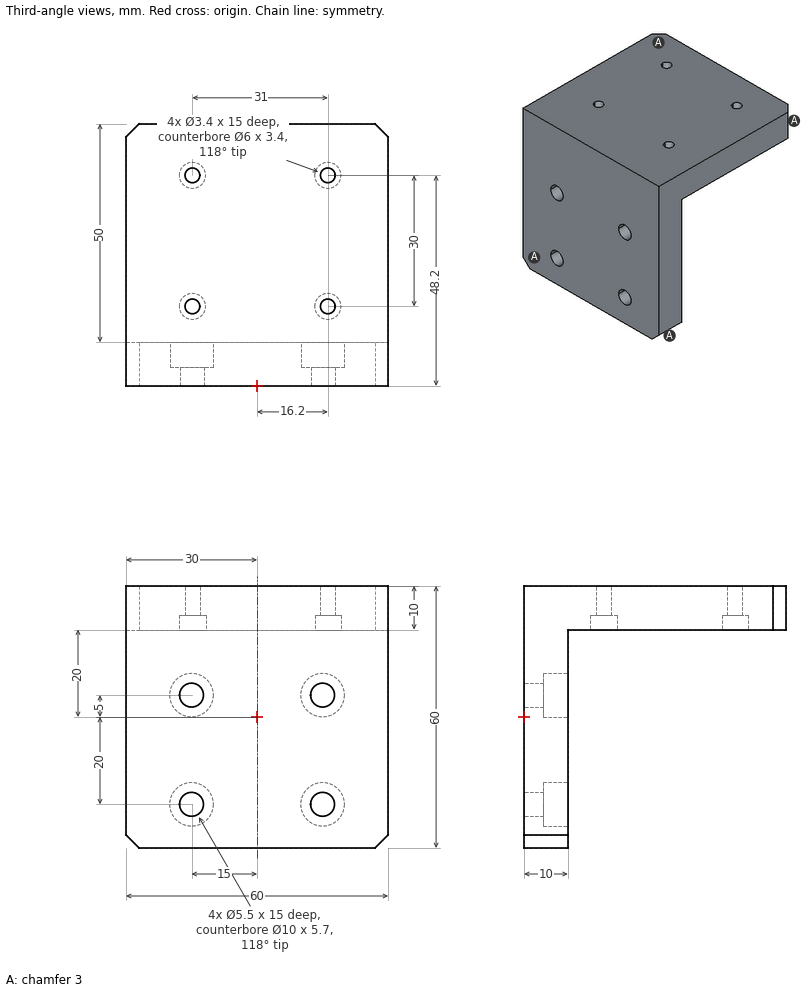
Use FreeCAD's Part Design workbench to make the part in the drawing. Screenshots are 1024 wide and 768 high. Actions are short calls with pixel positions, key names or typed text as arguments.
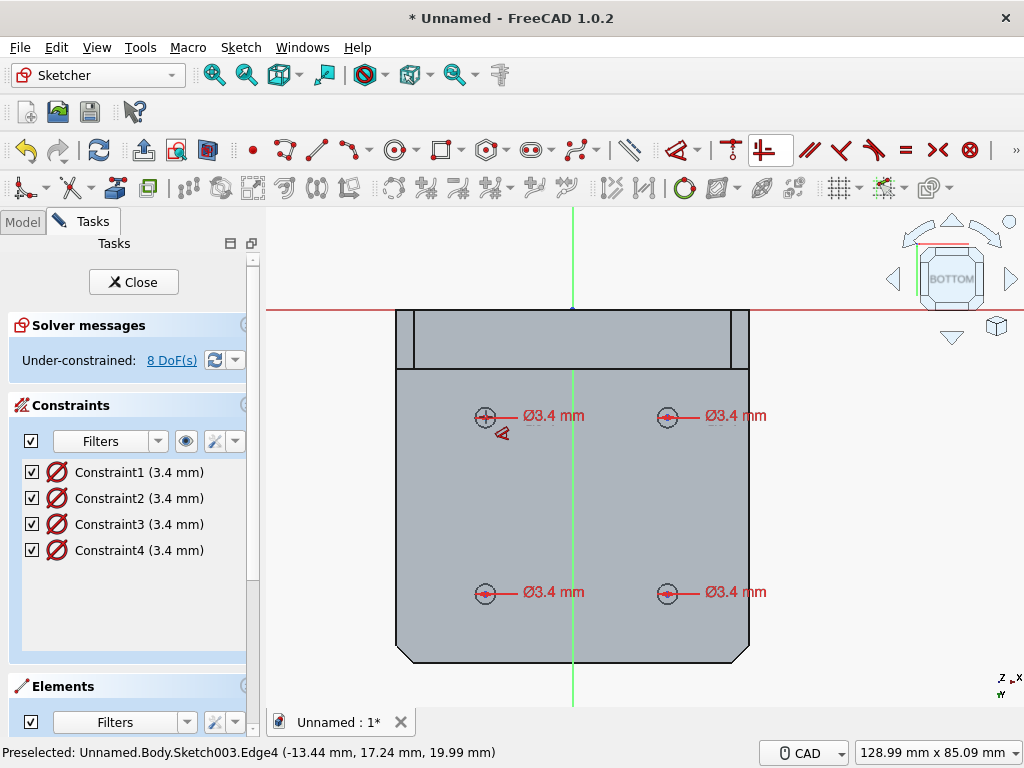
click(668, 594)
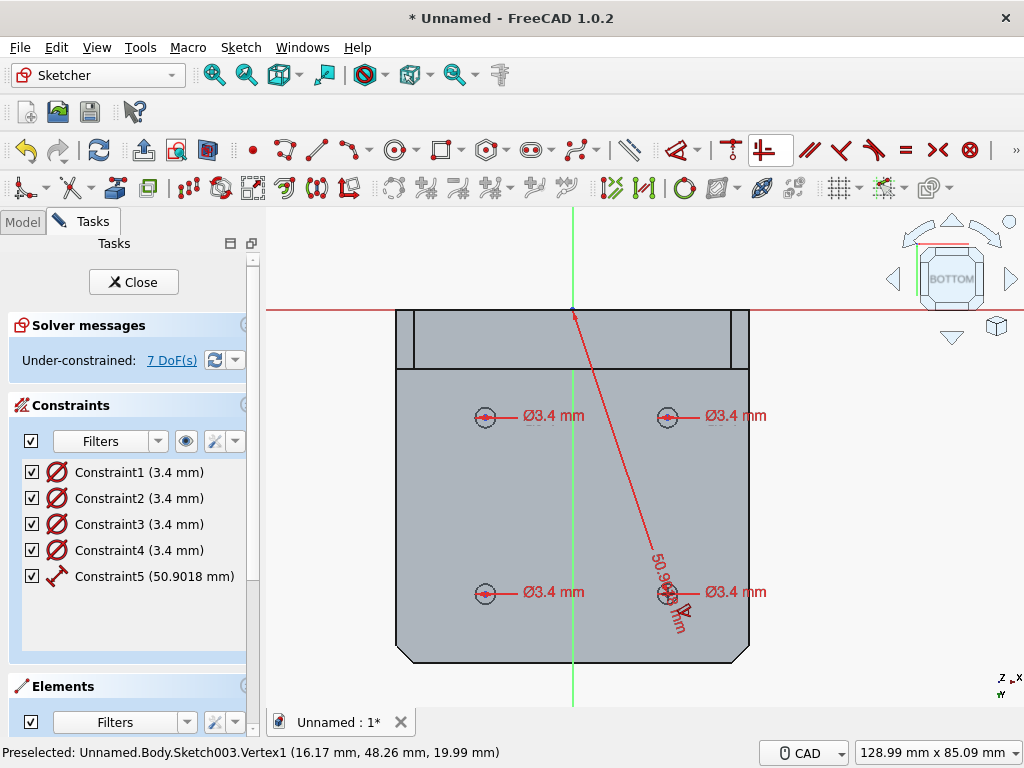
click(485, 594)
click(535, 628)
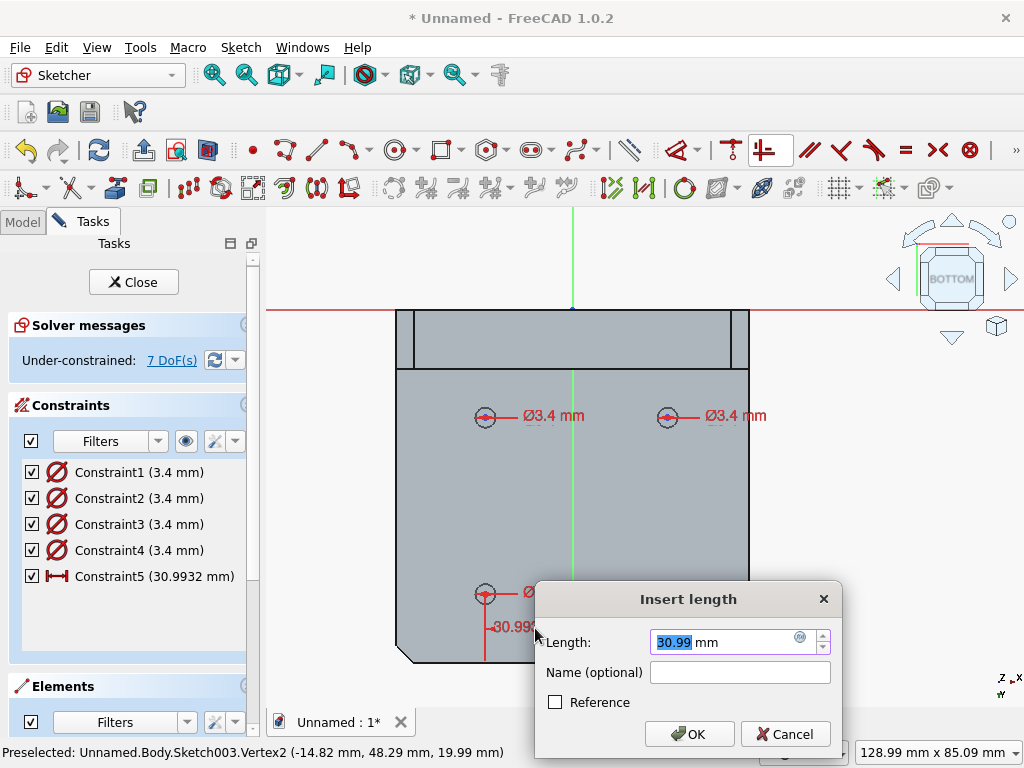
text(31)
key(Return)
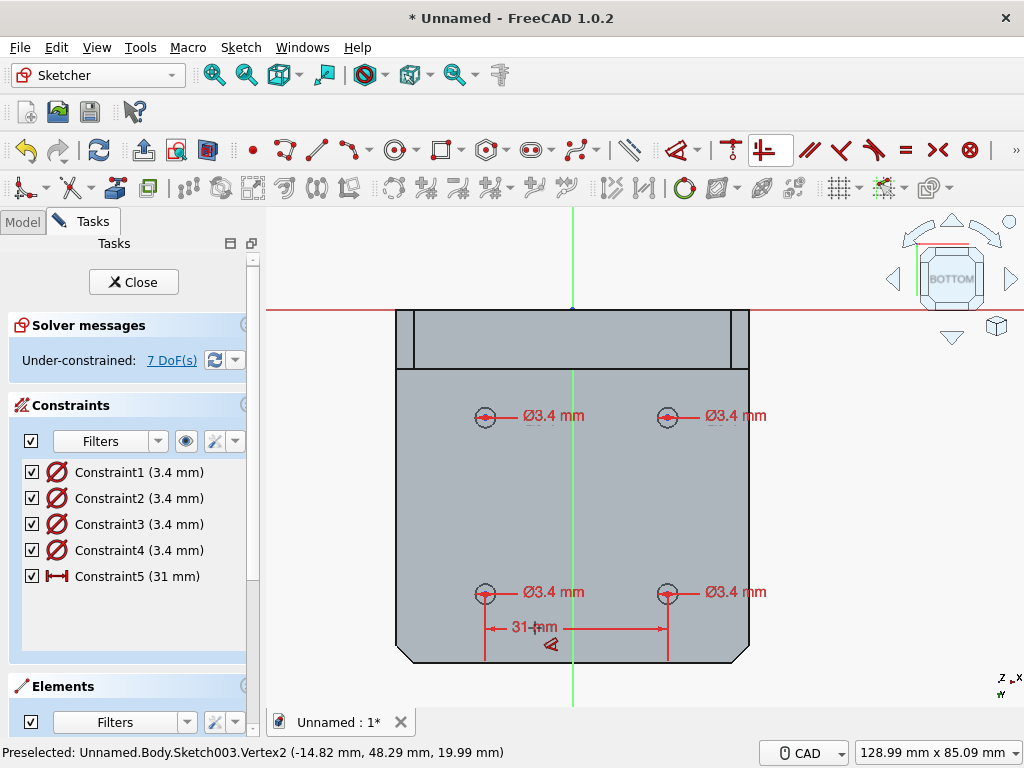
click(485, 594)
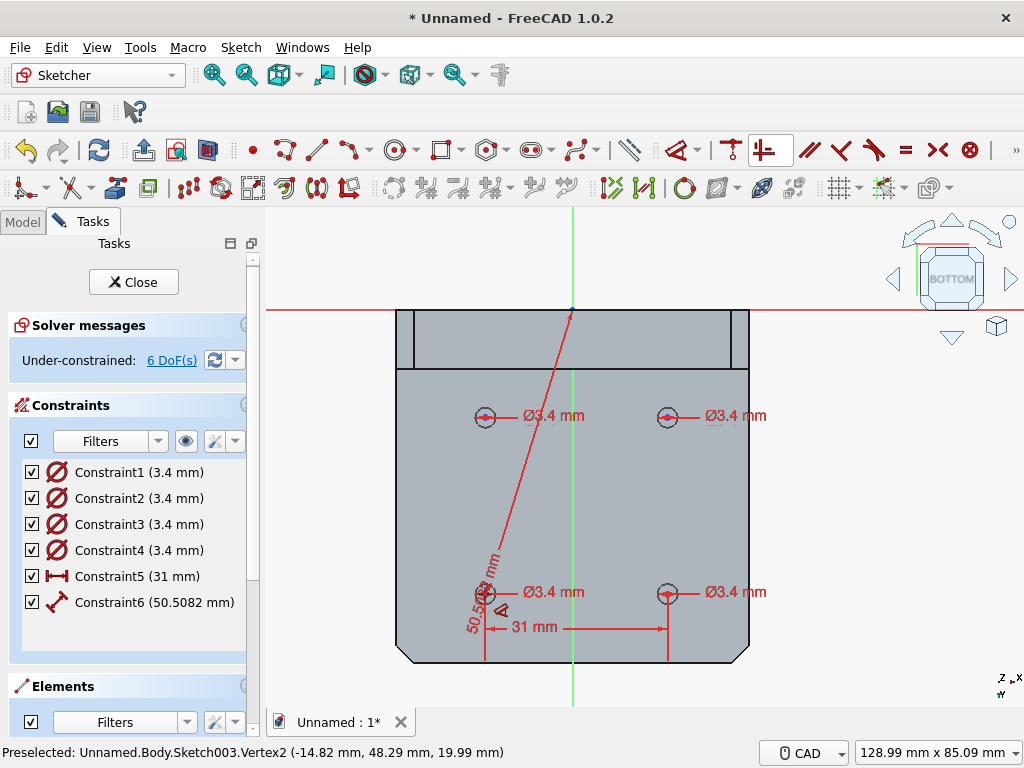
click(668, 418)
click(618, 628)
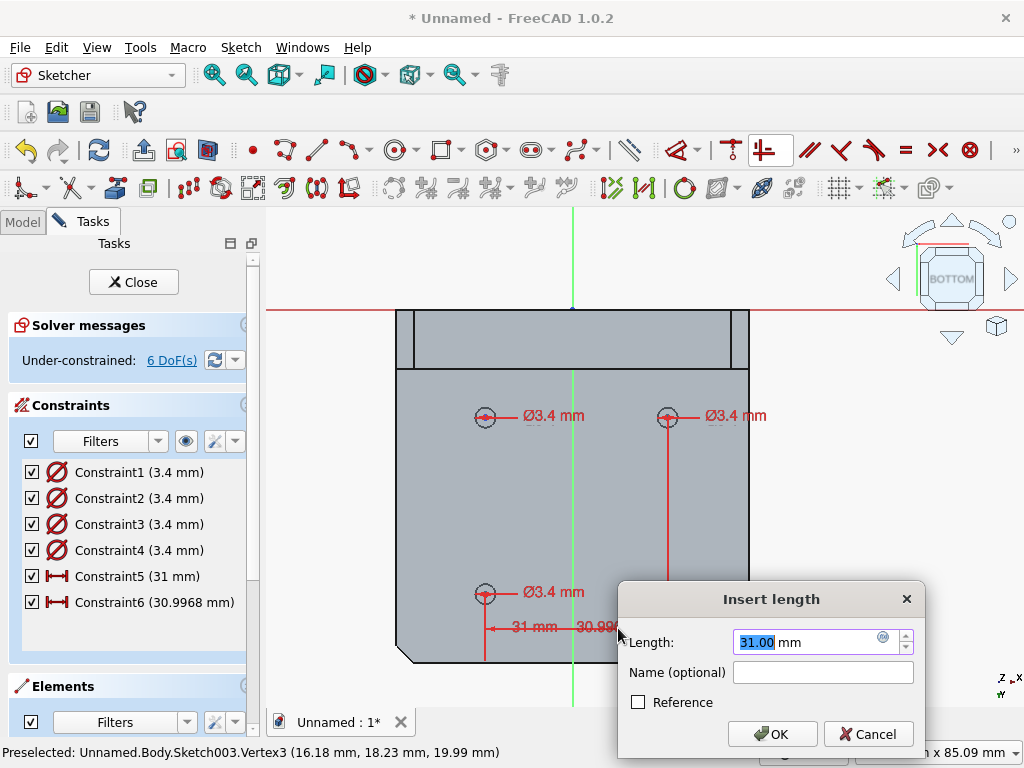
text(31)
key(Return)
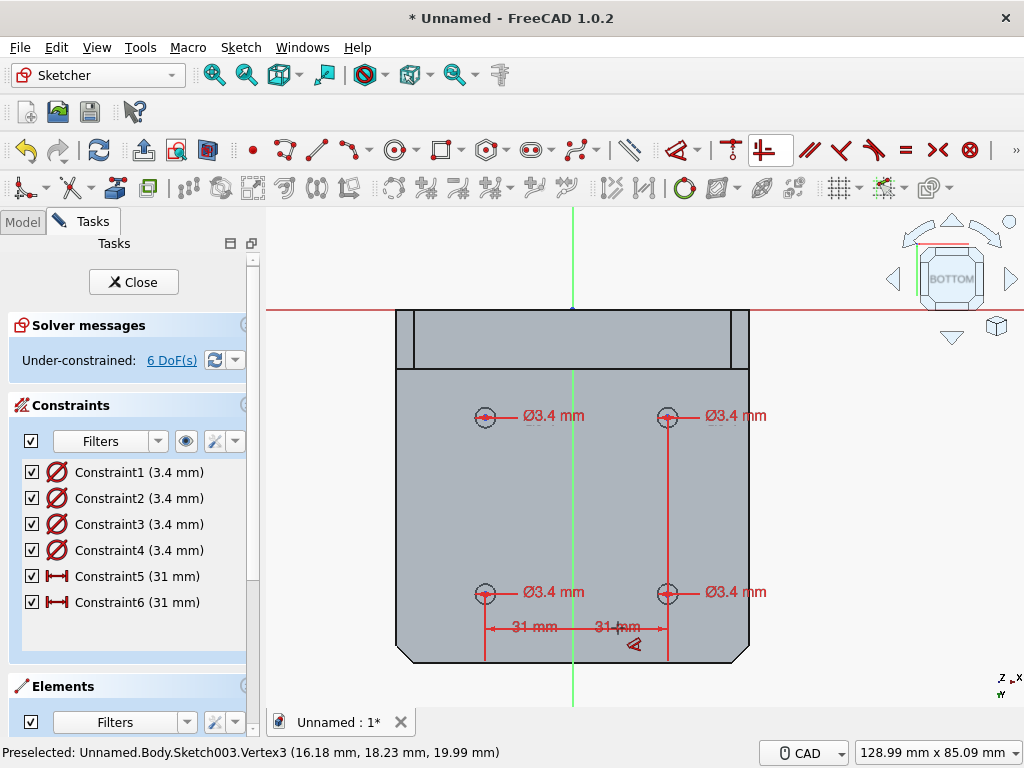
click(668, 594)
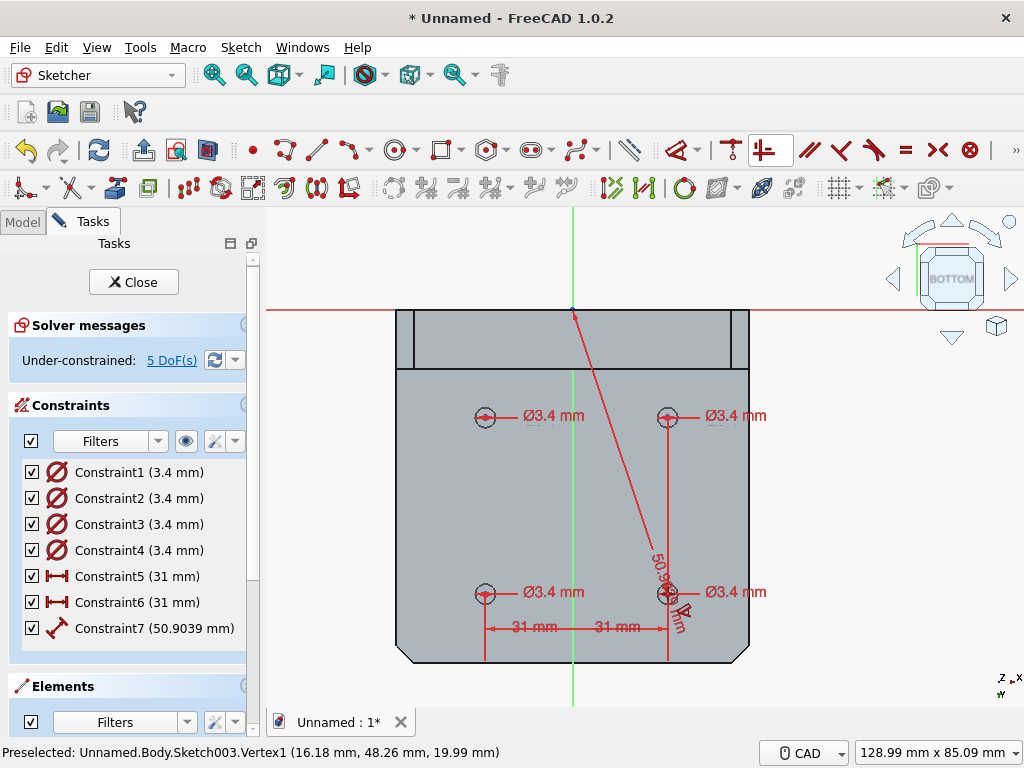
click(668, 418)
click(702, 506)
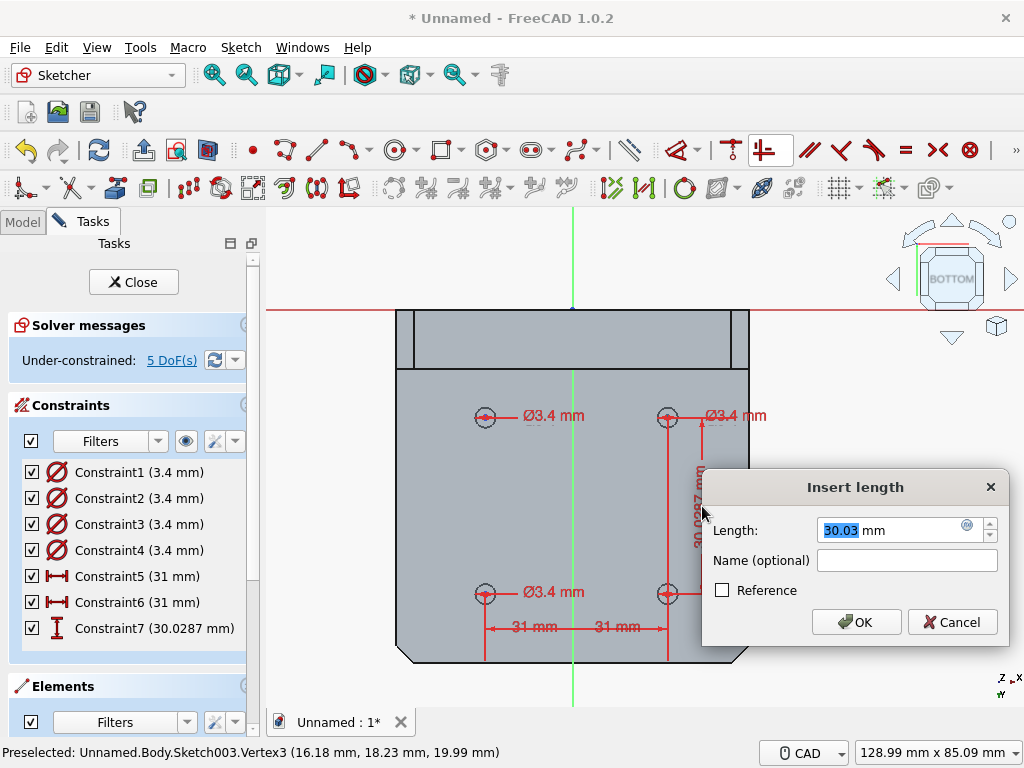
text(30)
key(Return)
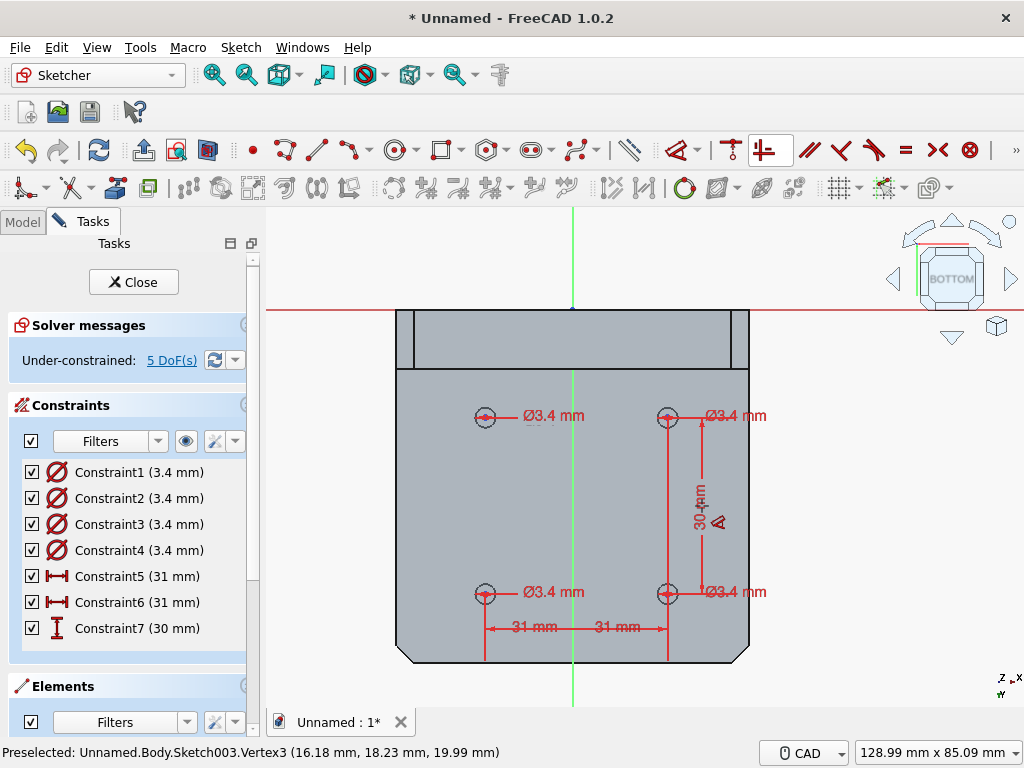
click(485, 594)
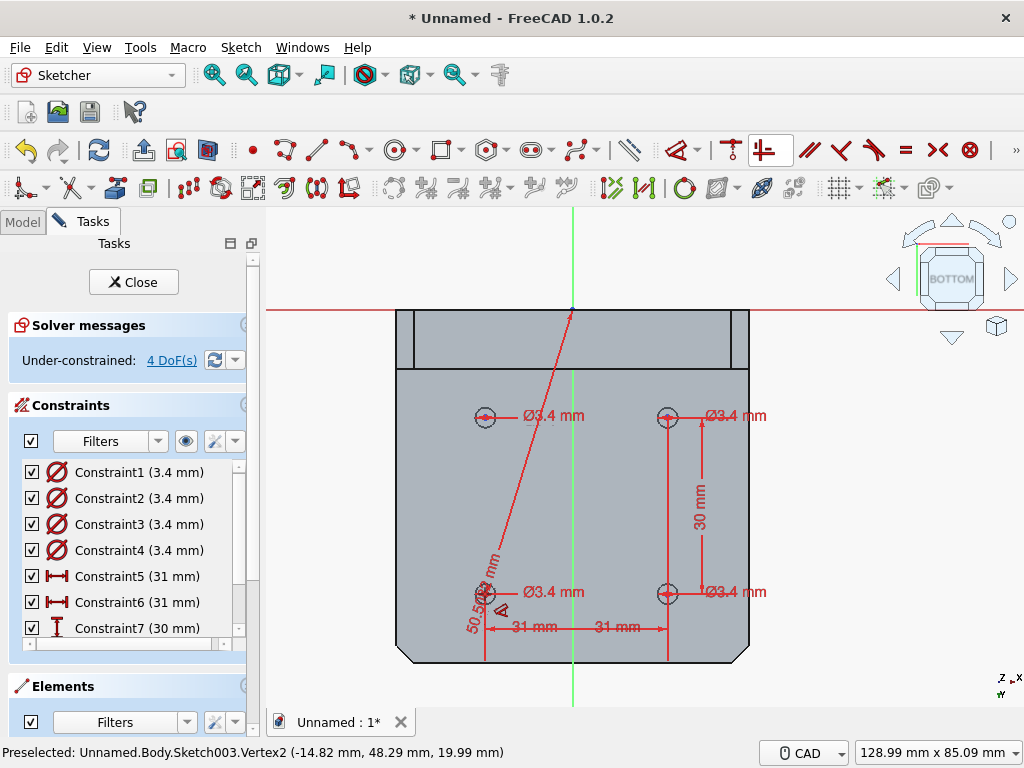
click(668, 418)
click(451, 506)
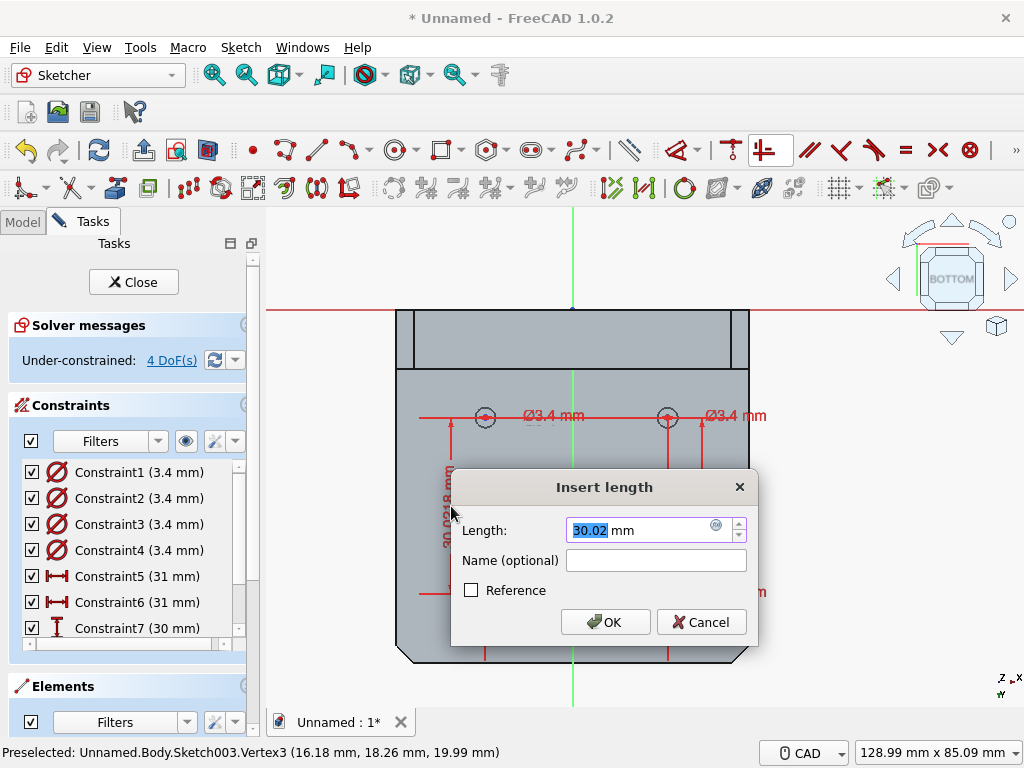
text(30)
key(Return)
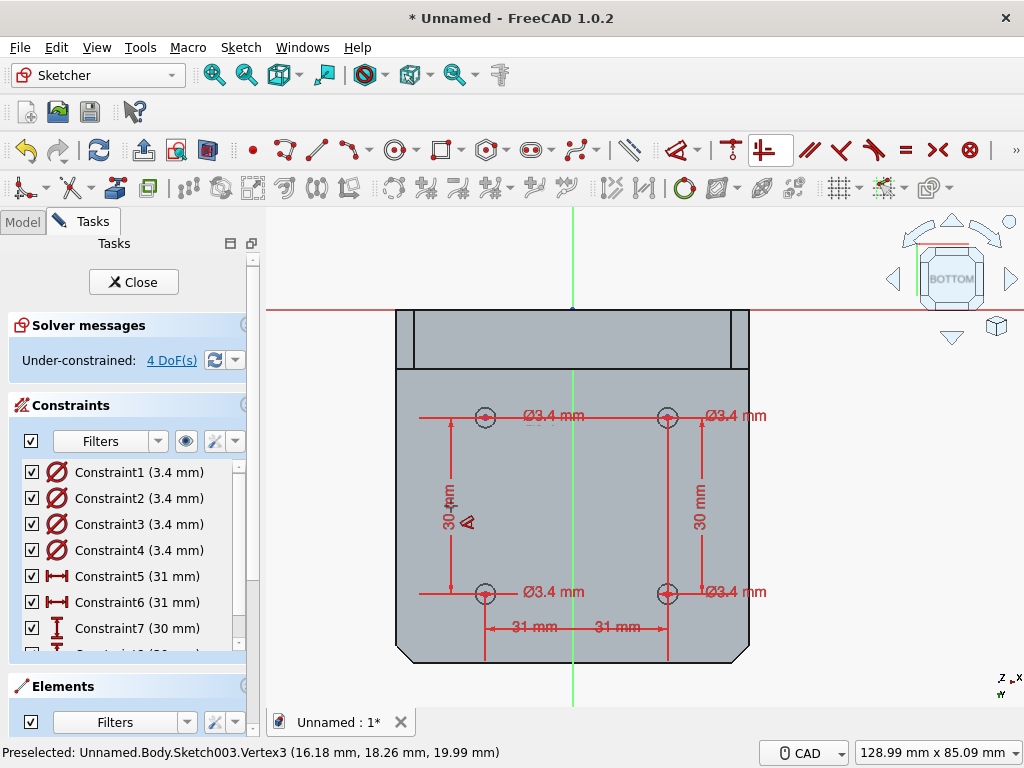
click(668, 418)